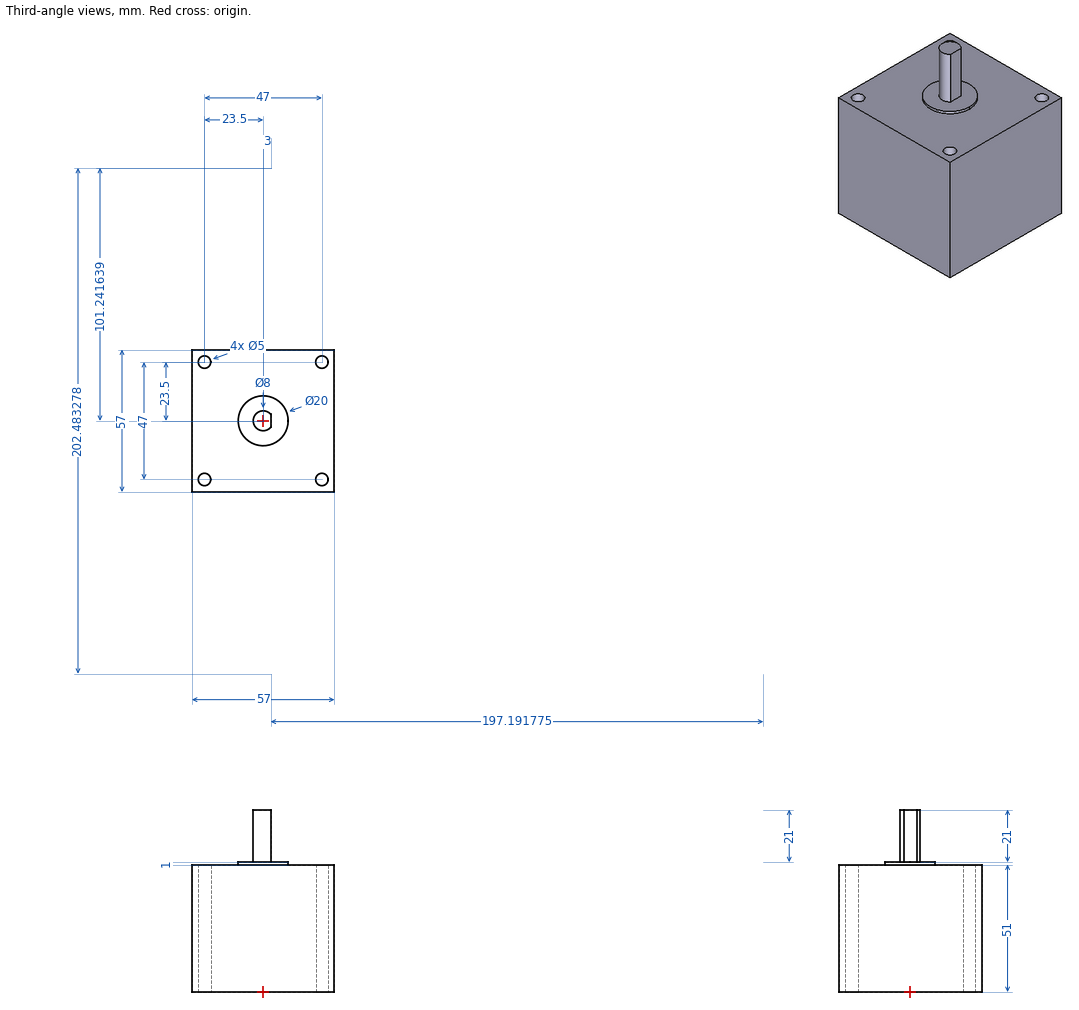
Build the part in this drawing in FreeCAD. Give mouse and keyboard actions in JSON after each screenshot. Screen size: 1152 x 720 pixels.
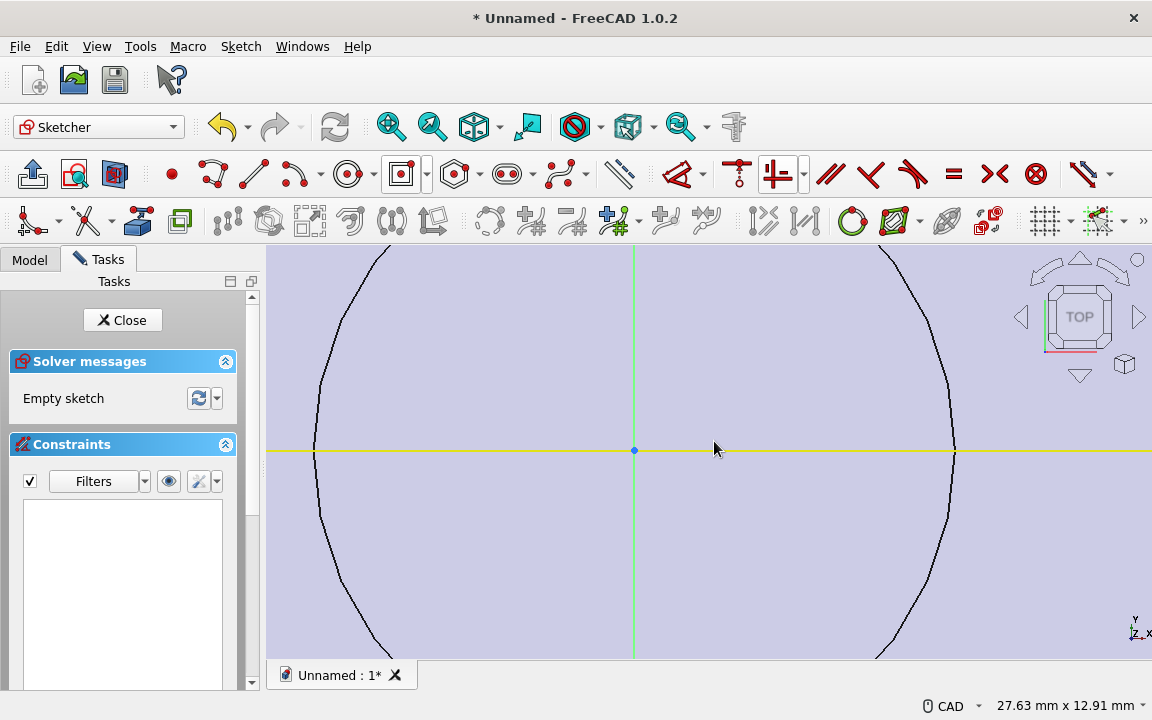
{"action": "left_click", "coordinate": [348, 174]}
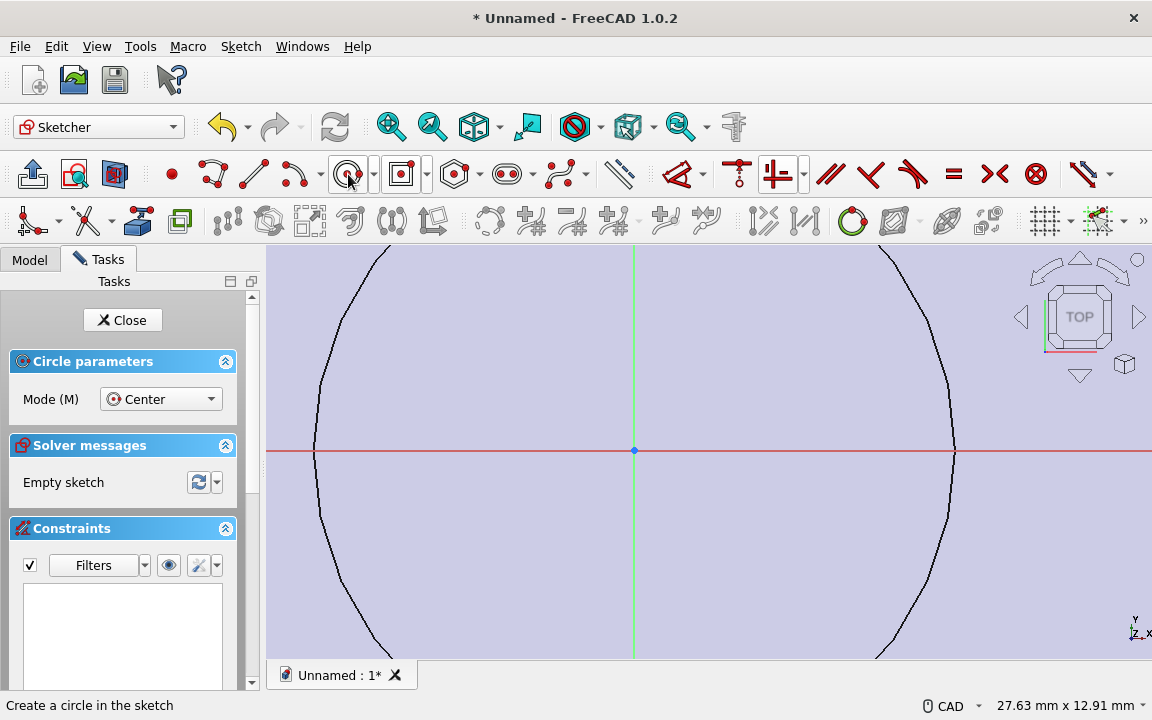
{"action": "left_click", "coordinate": [634, 451]}
{"action": "left_click", "coordinate": [725, 360]}
{"action": "key", "text": "Escape"}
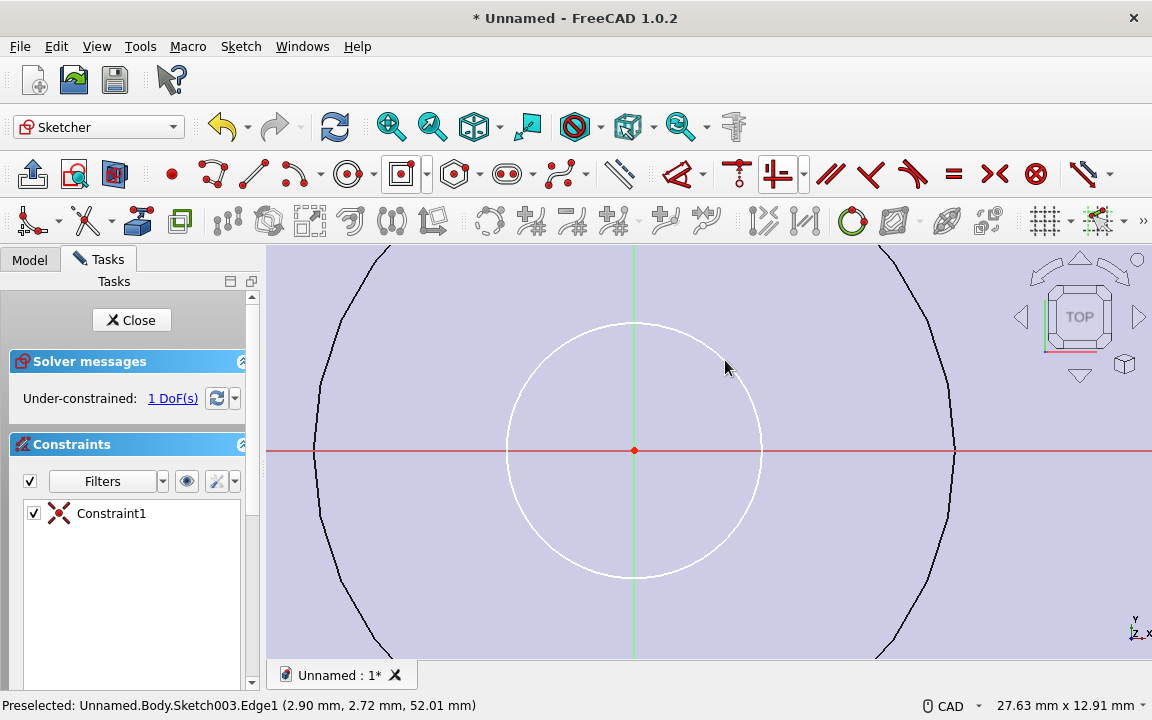
{"action": "left_click", "coordinate": [676, 174]}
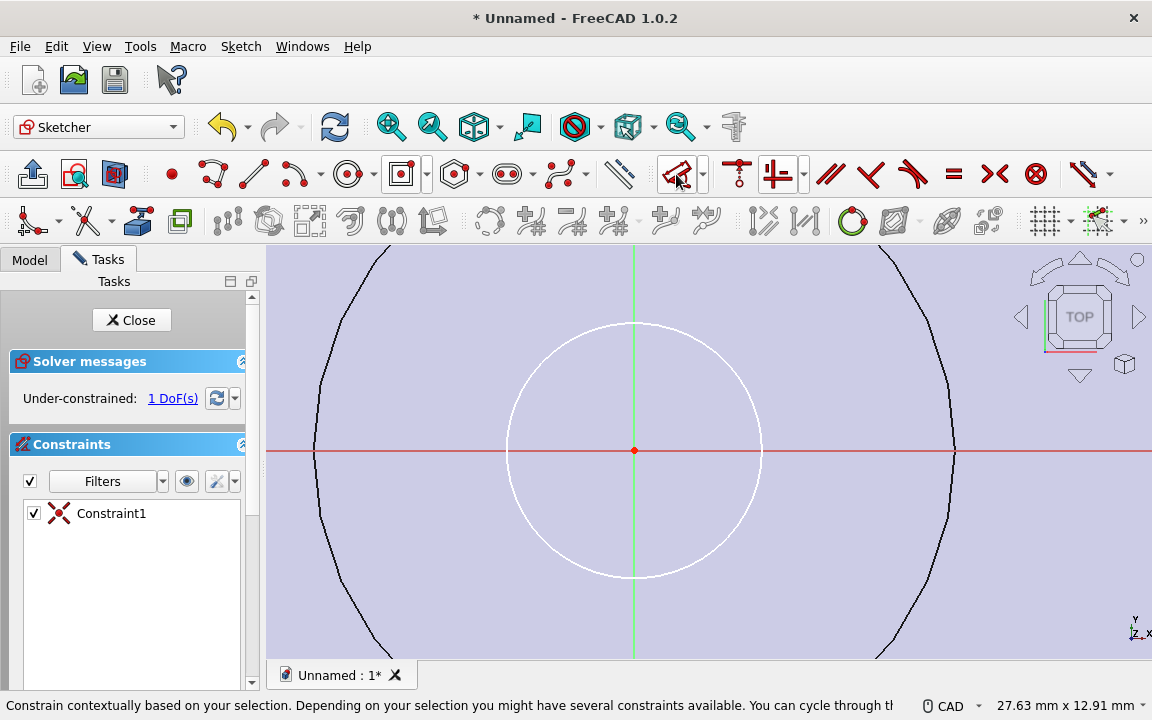
{"action": "left_click", "coordinate": [724, 360]}
{"action": "left_click", "coordinate": [746, 337]}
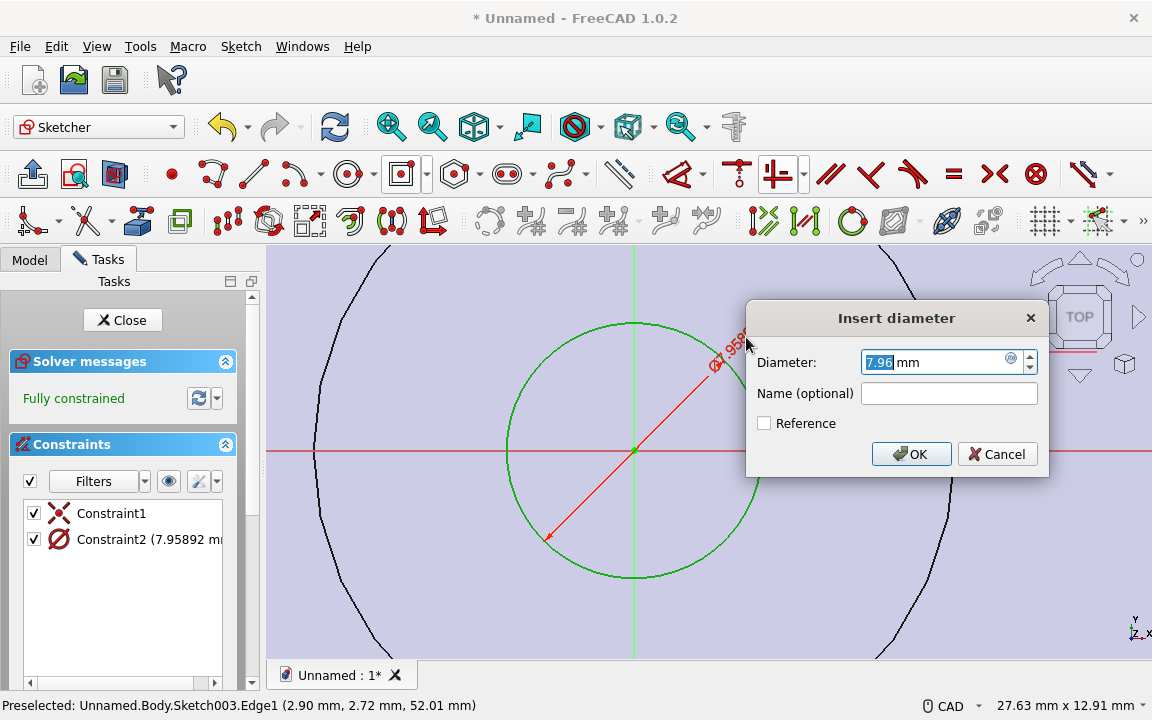
{"action": "type", "text": "8"}
{"action": "key", "text": "Return"}
{"action": "key", "text": "Escape"}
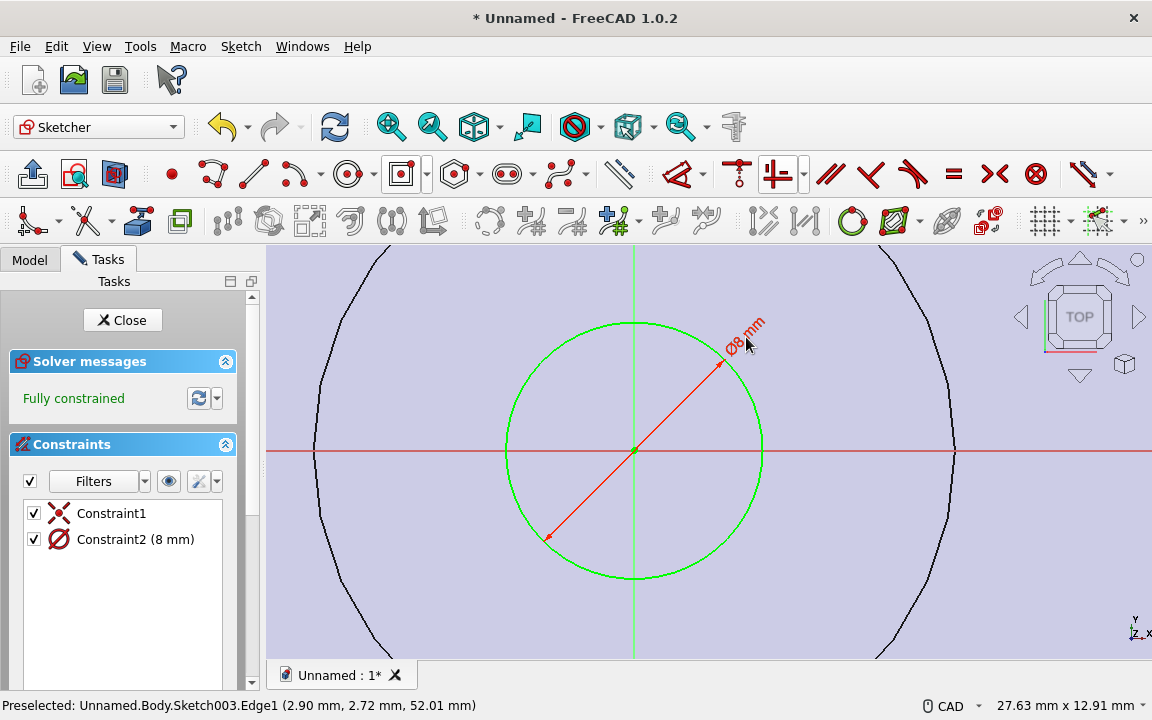
{"action": "left_click", "coordinate": [123, 320]}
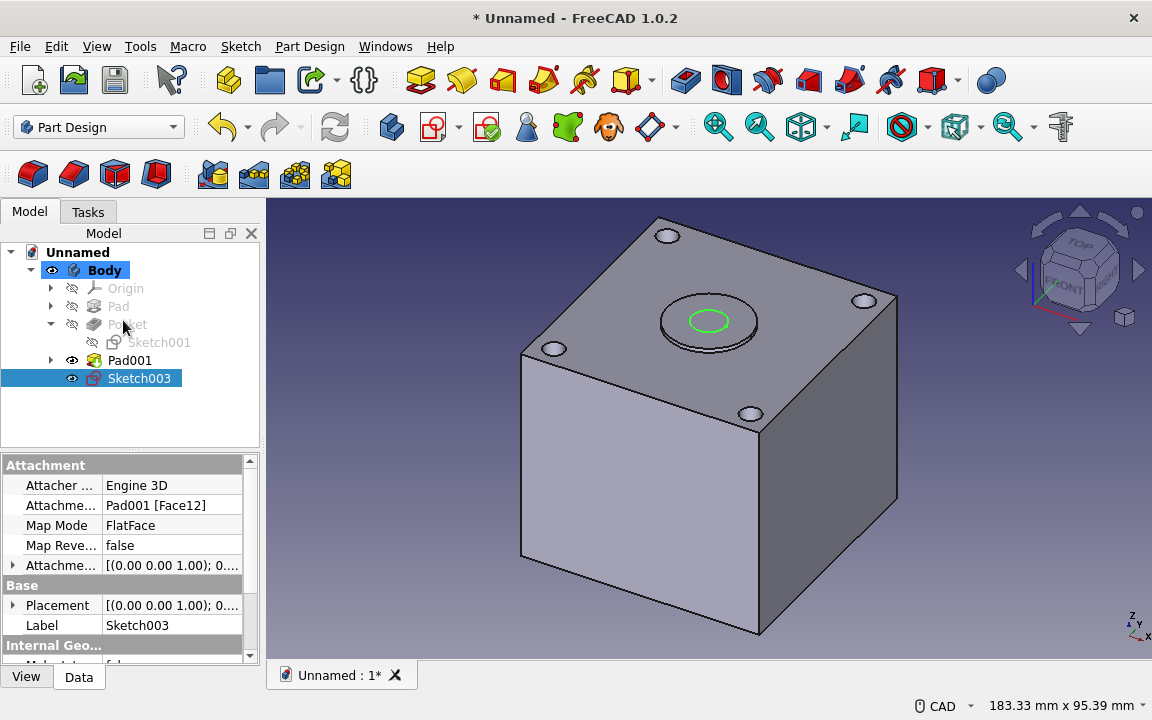
{"action": "left_click", "coordinate": [421, 80]}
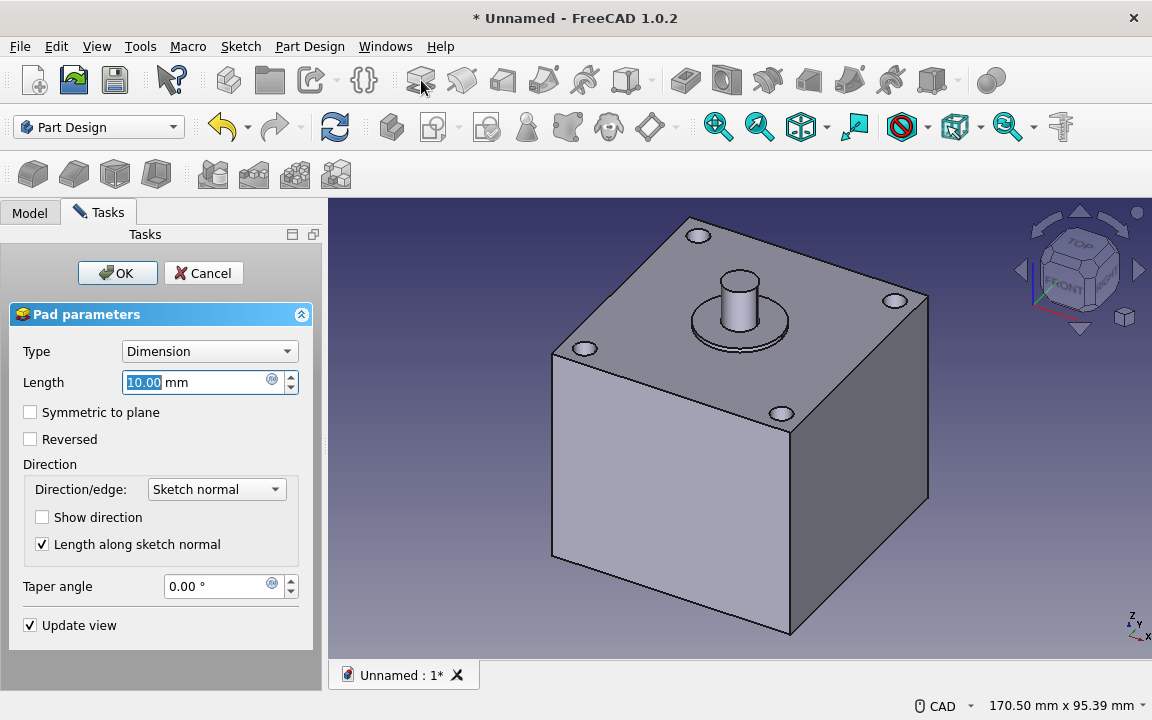
{"action": "type", "text": "21"}
{"action": "key", "text": "Tab"}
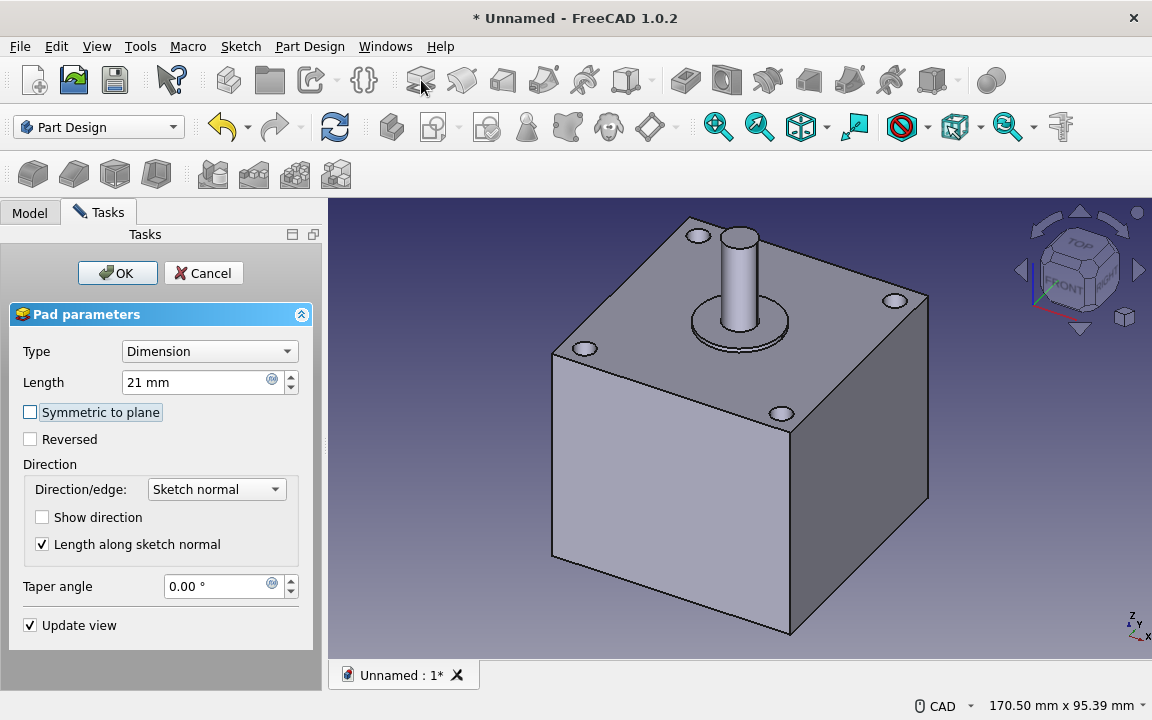
{"action": "left_click", "coordinate": [118, 273]}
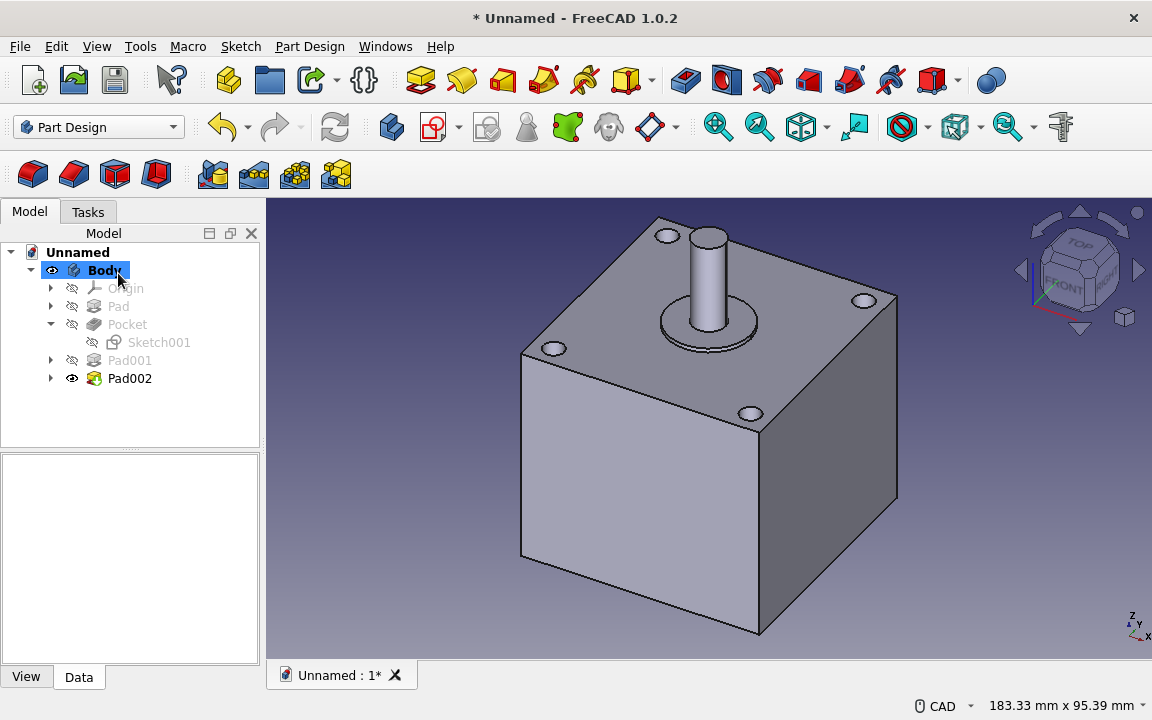
{"action": "left_click", "coordinate": [719, 128]}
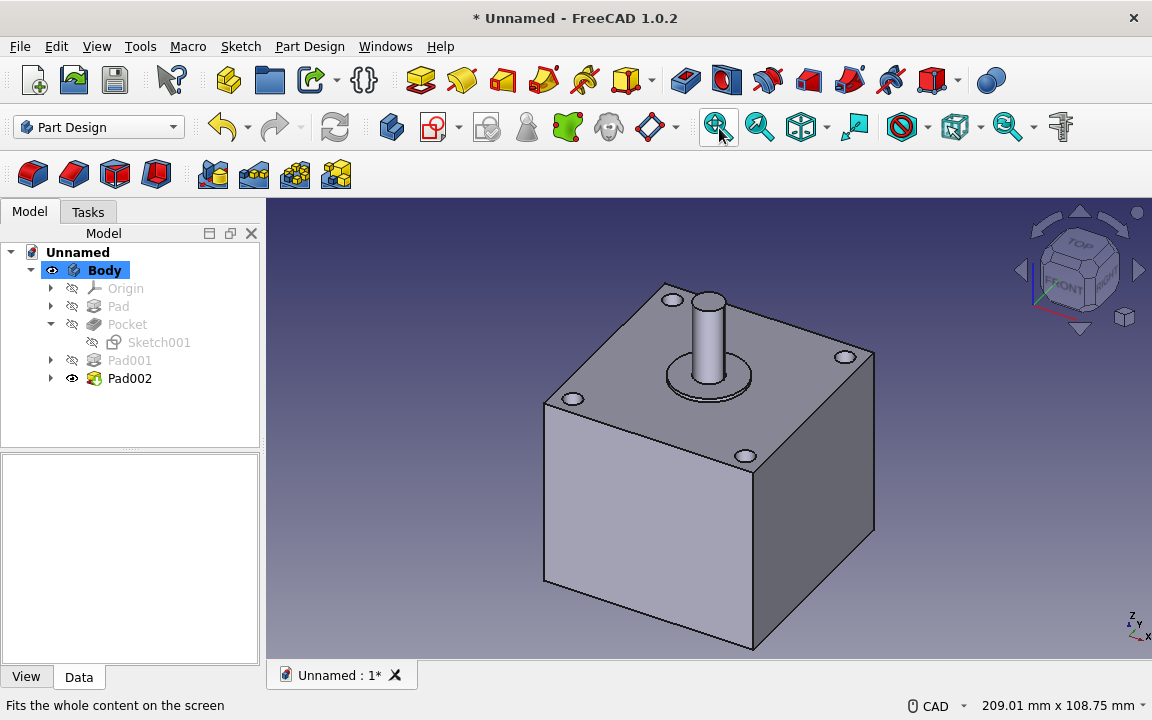
{"action": "left_click", "coordinate": [709, 301]}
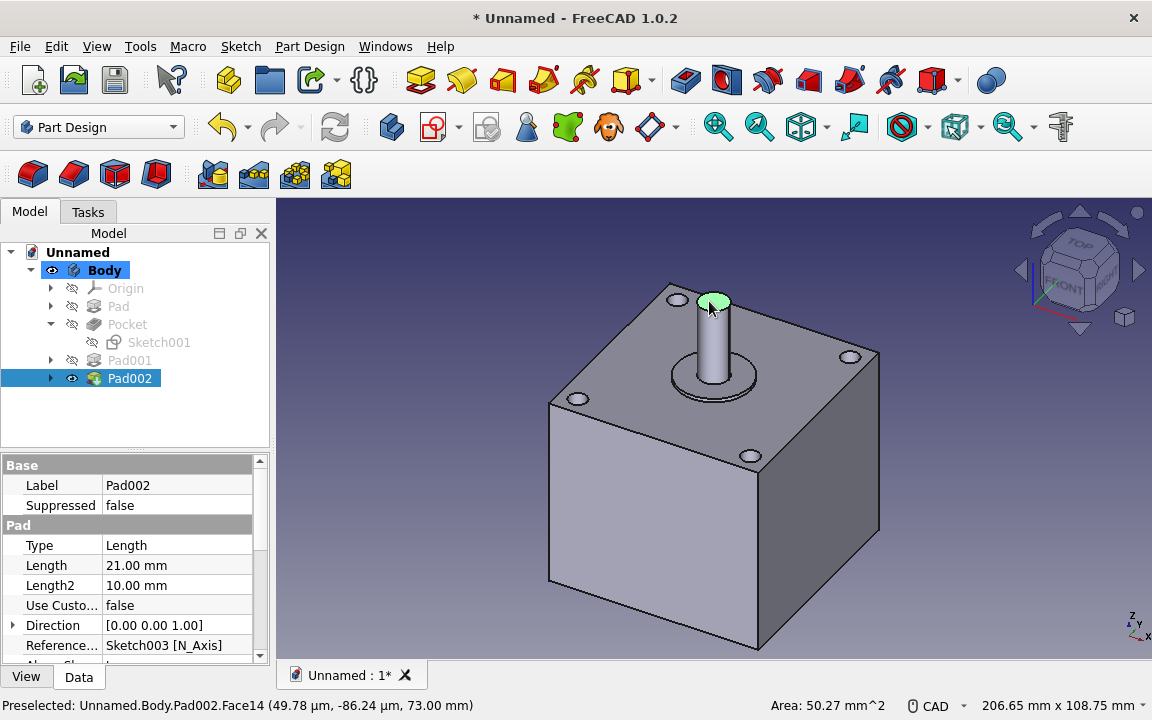
{"action": "left_click", "coordinate": [432, 128]}